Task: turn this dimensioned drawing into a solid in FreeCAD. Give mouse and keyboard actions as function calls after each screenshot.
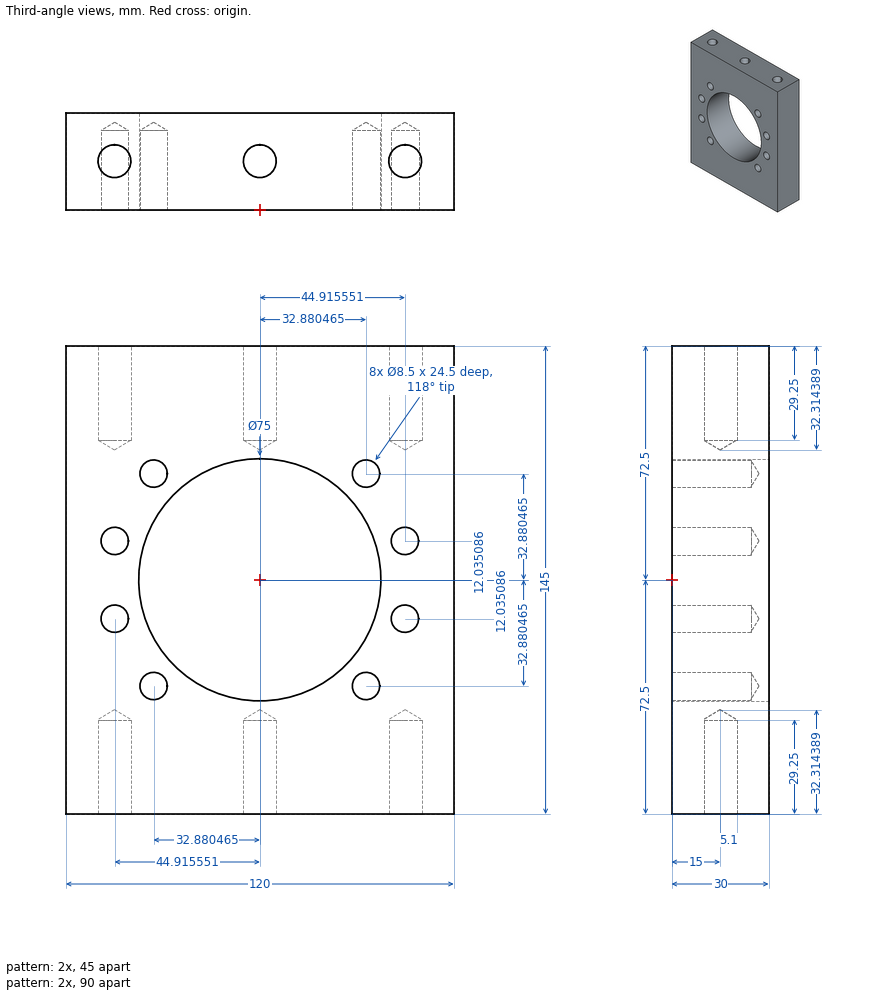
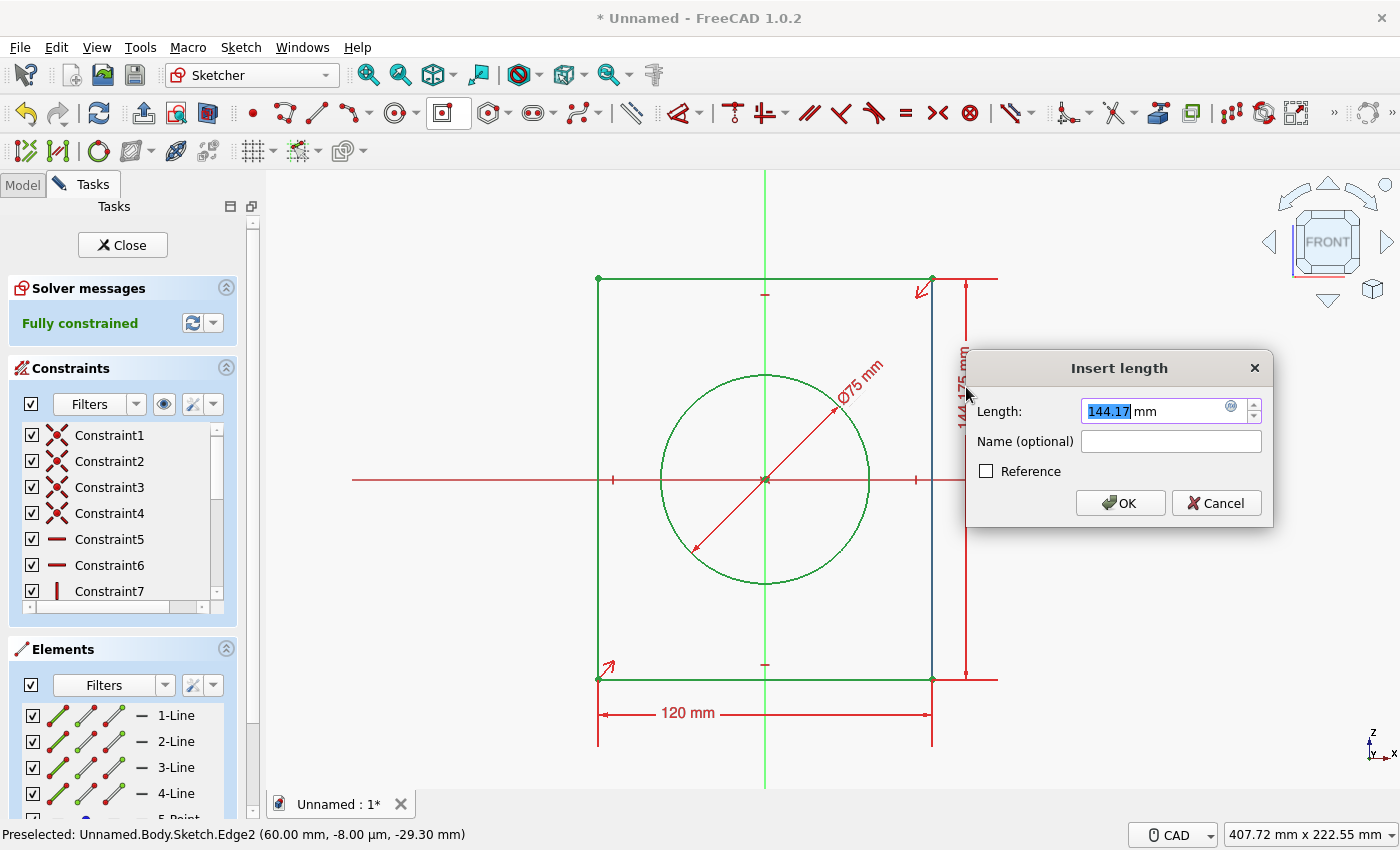
text(145)
key(Return)
key(Escape)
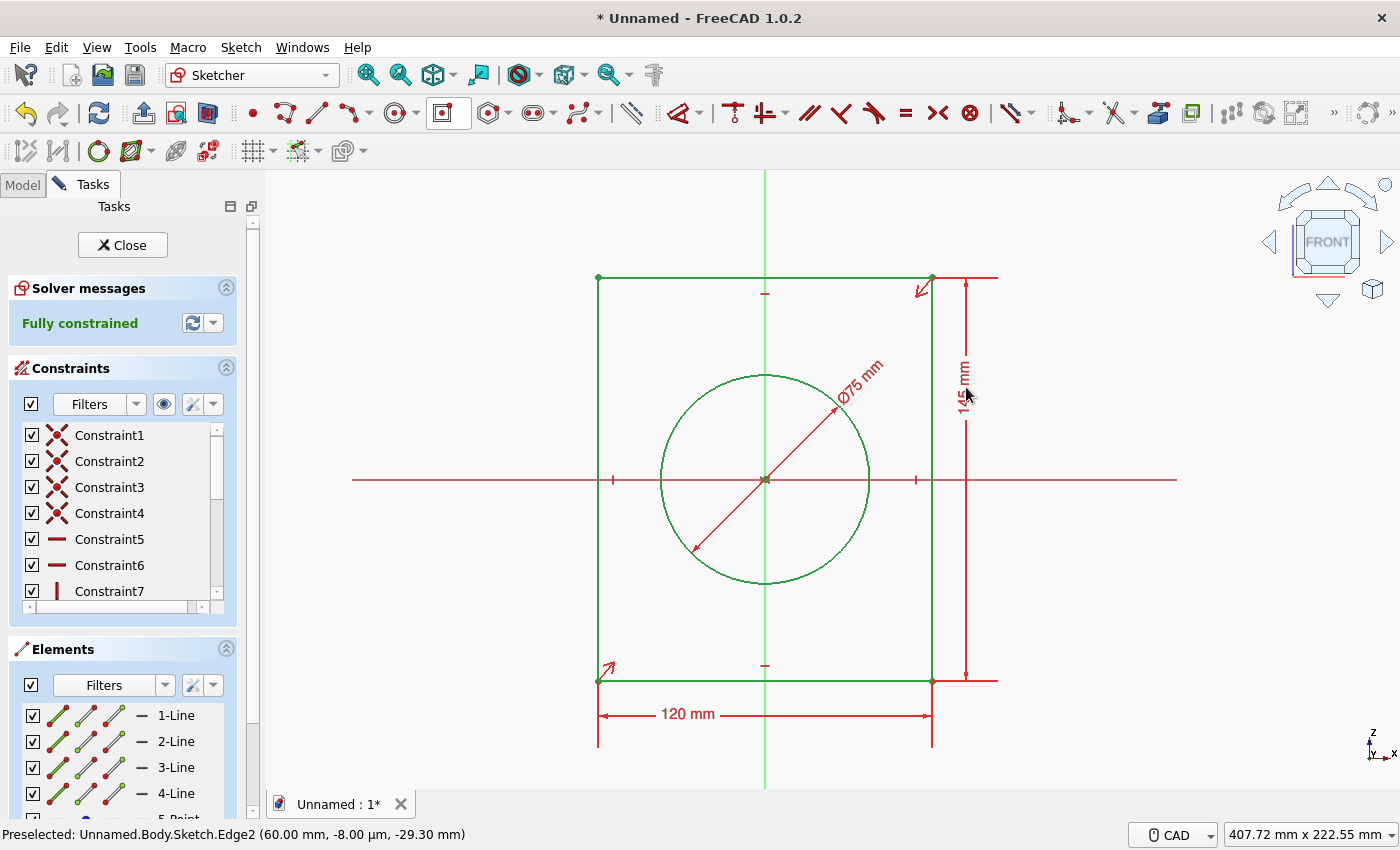
click(123, 245)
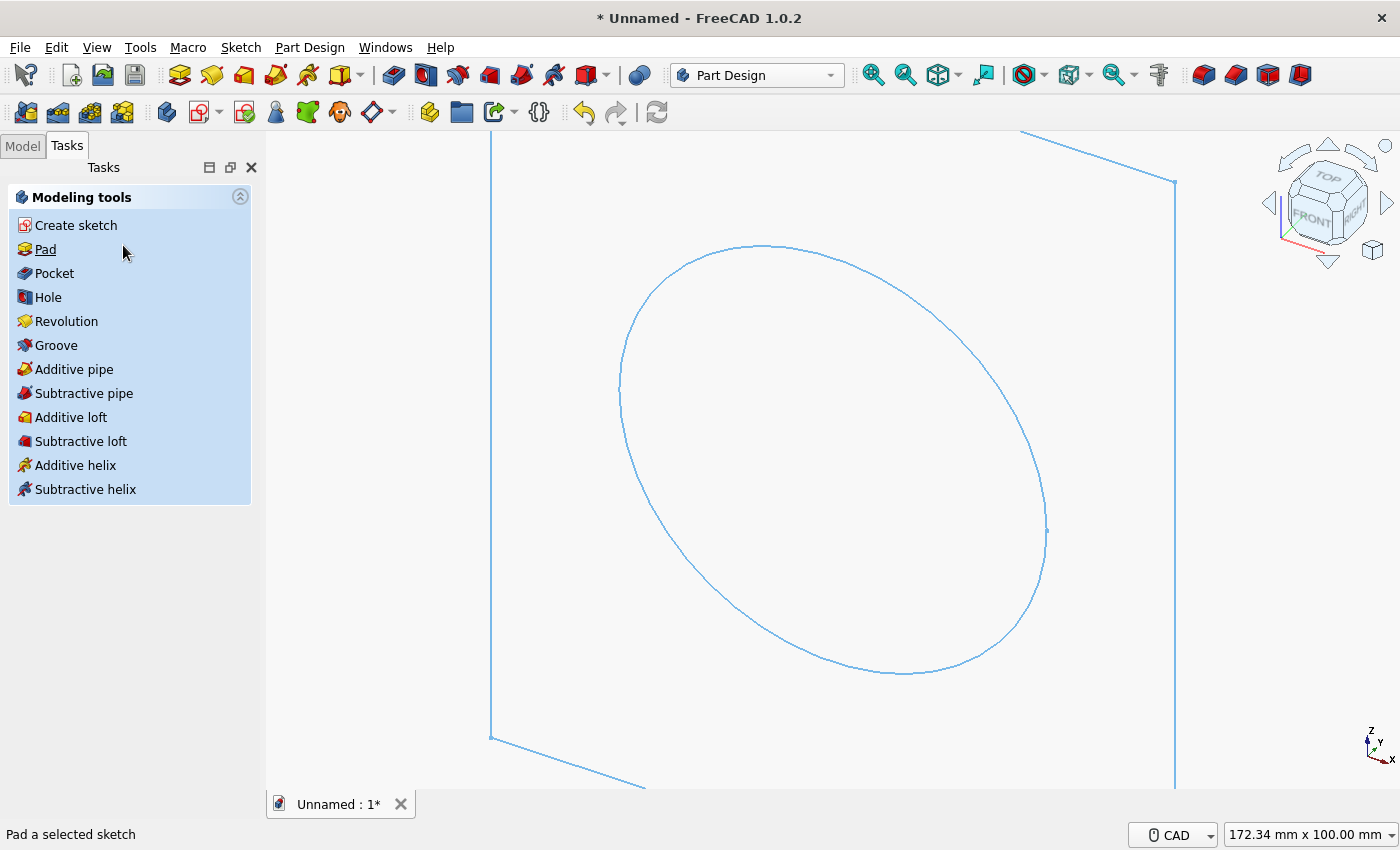
click(180, 76)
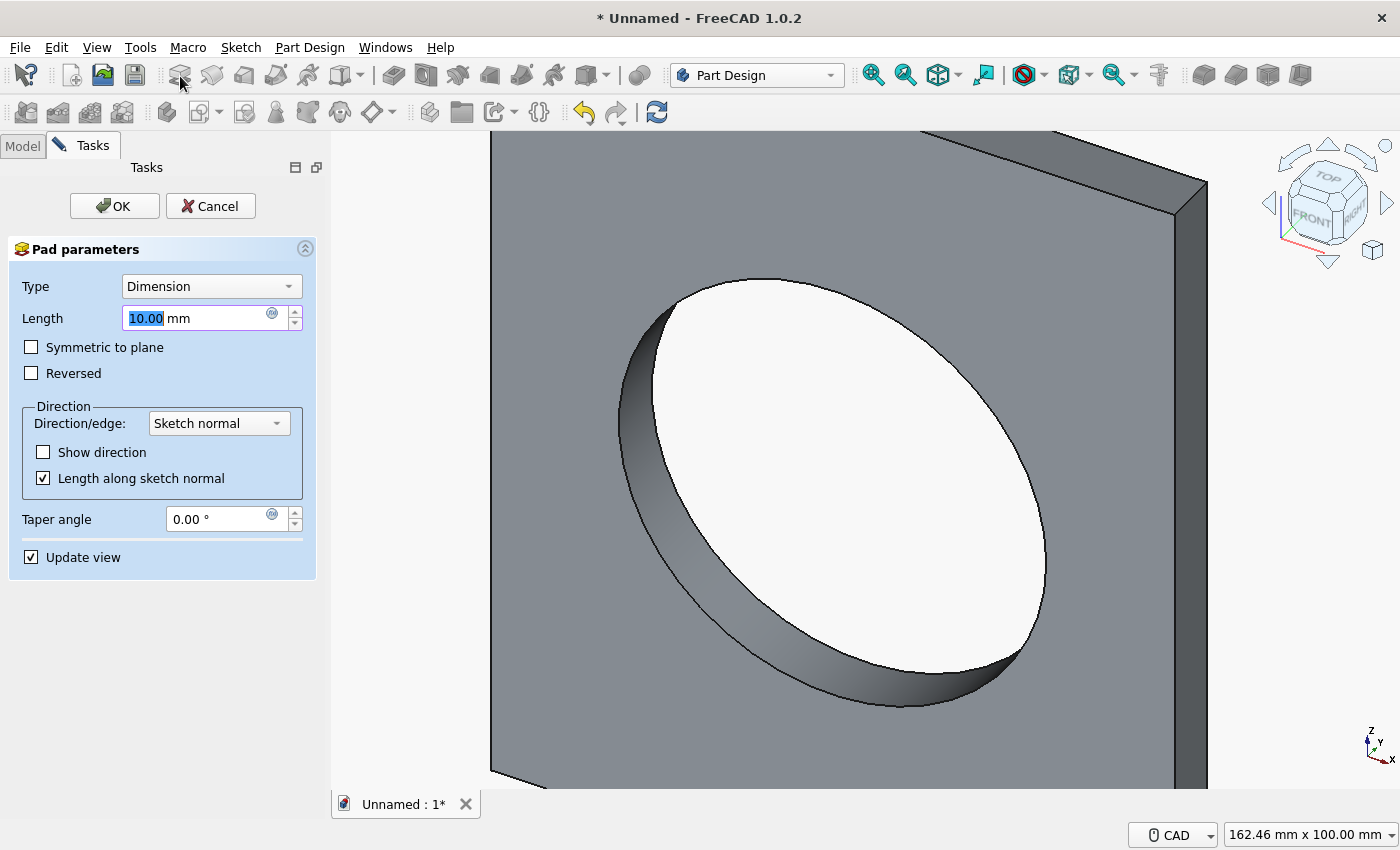
text(30)
key(Tab)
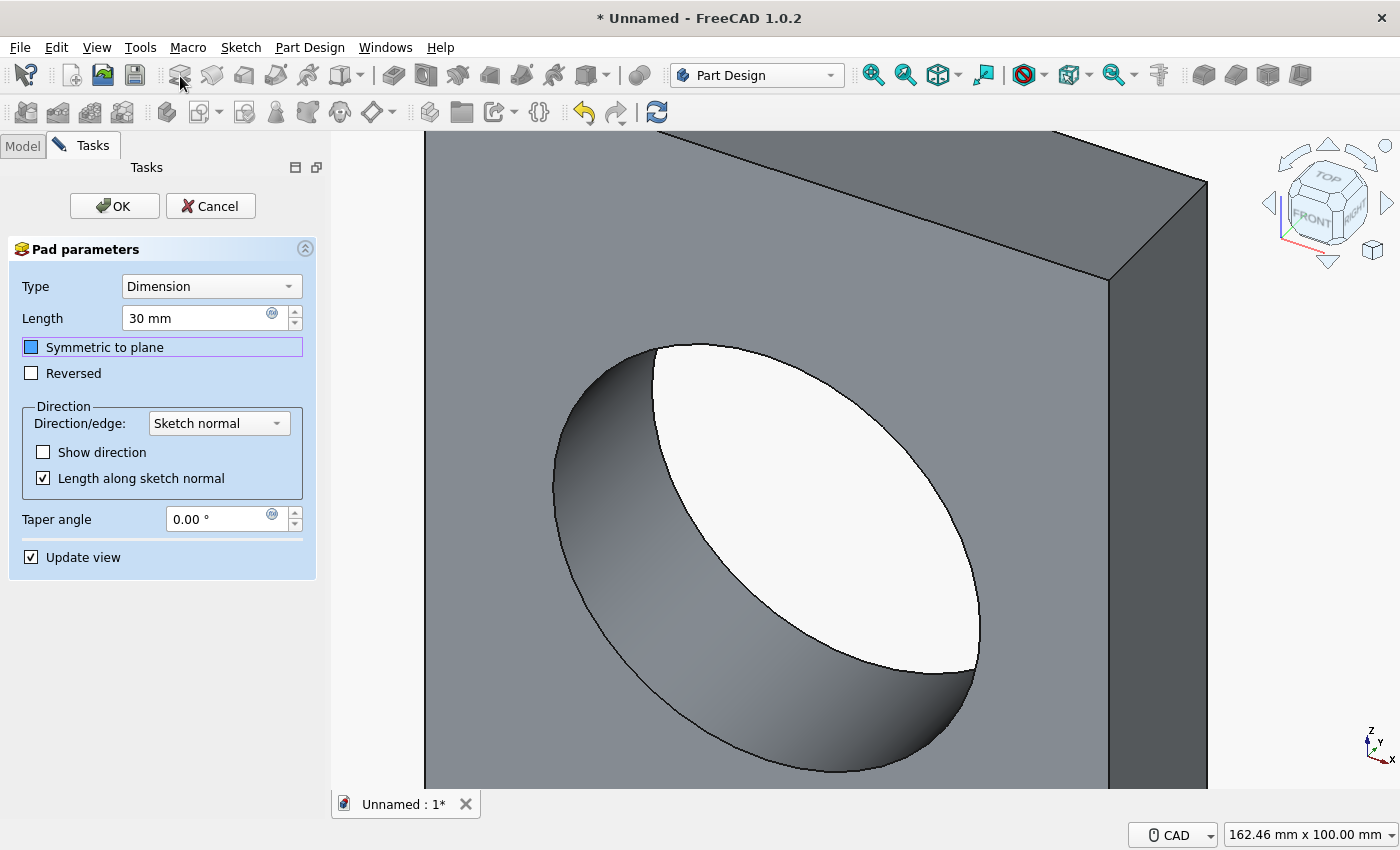
click(30, 373)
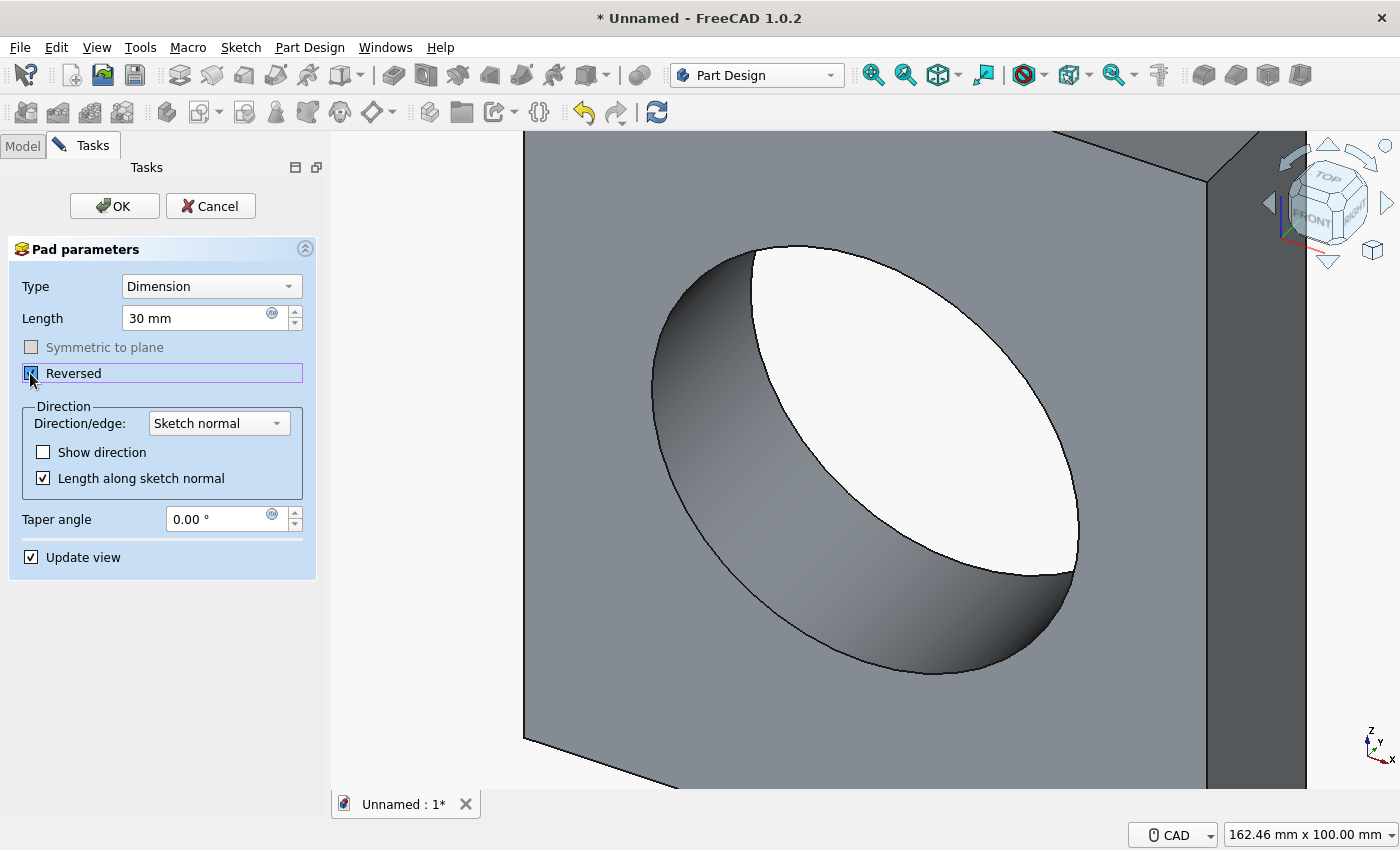
click(115, 206)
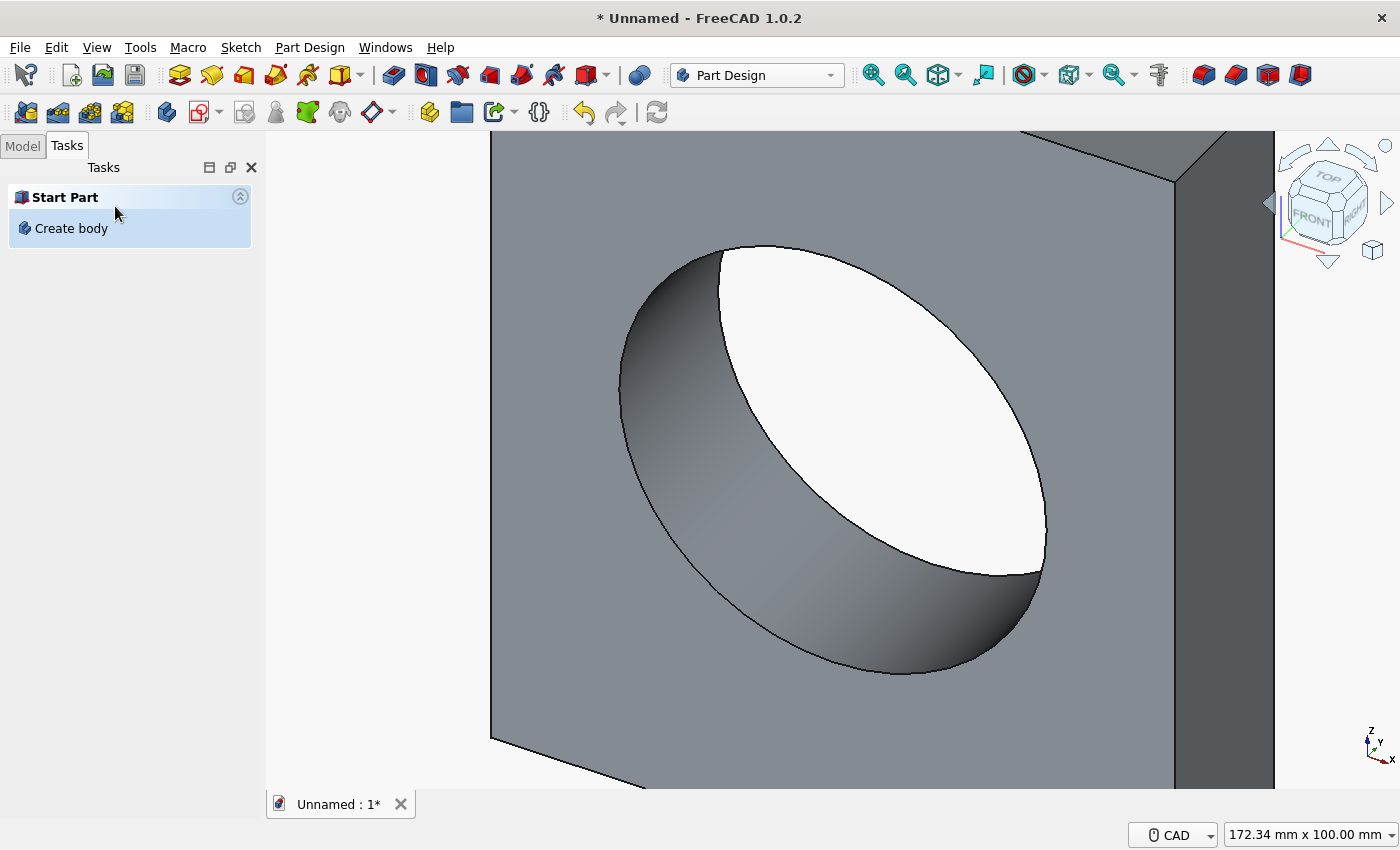
click(874, 76)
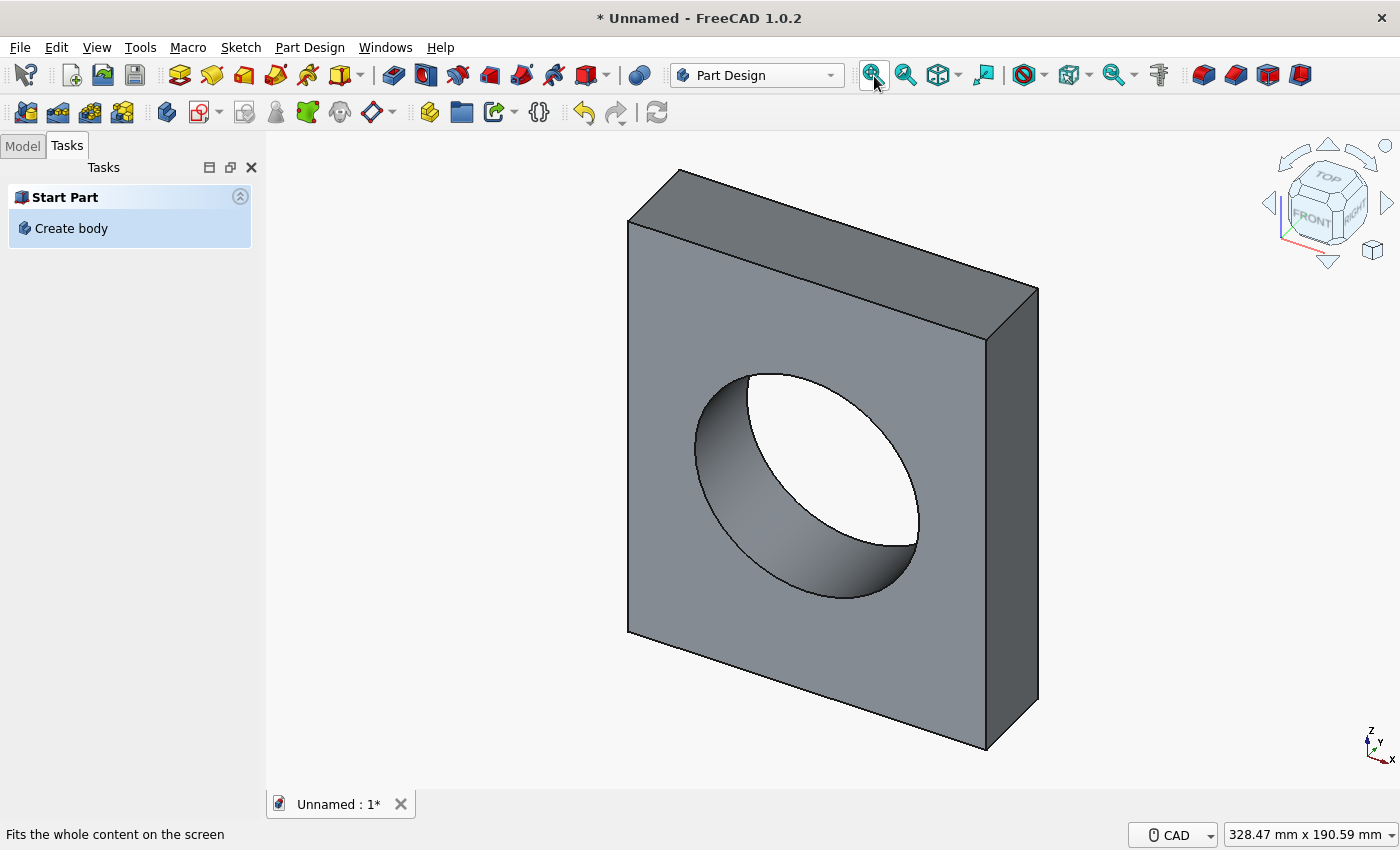
click(200, 112)